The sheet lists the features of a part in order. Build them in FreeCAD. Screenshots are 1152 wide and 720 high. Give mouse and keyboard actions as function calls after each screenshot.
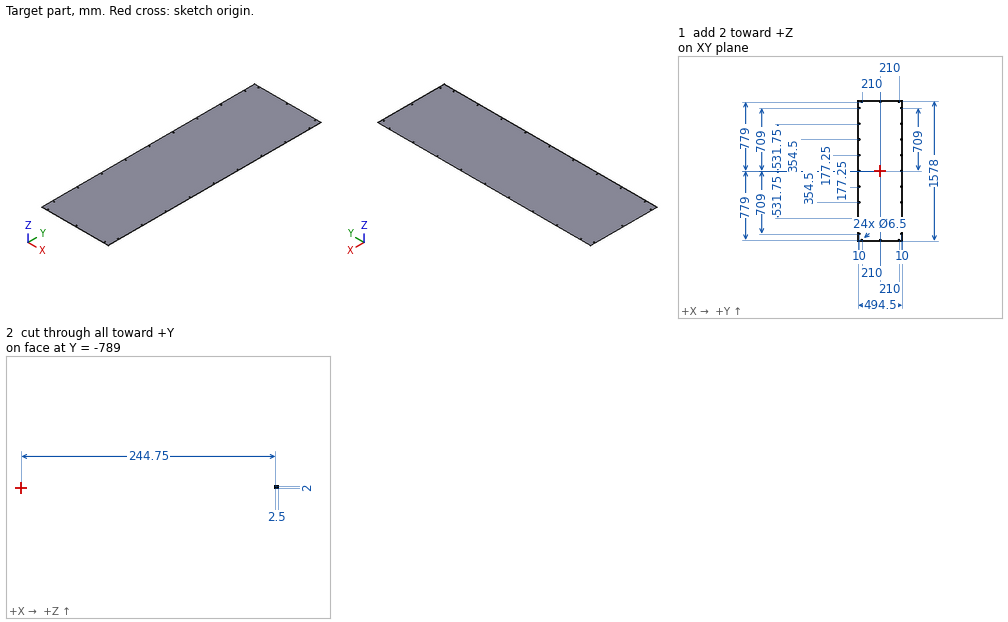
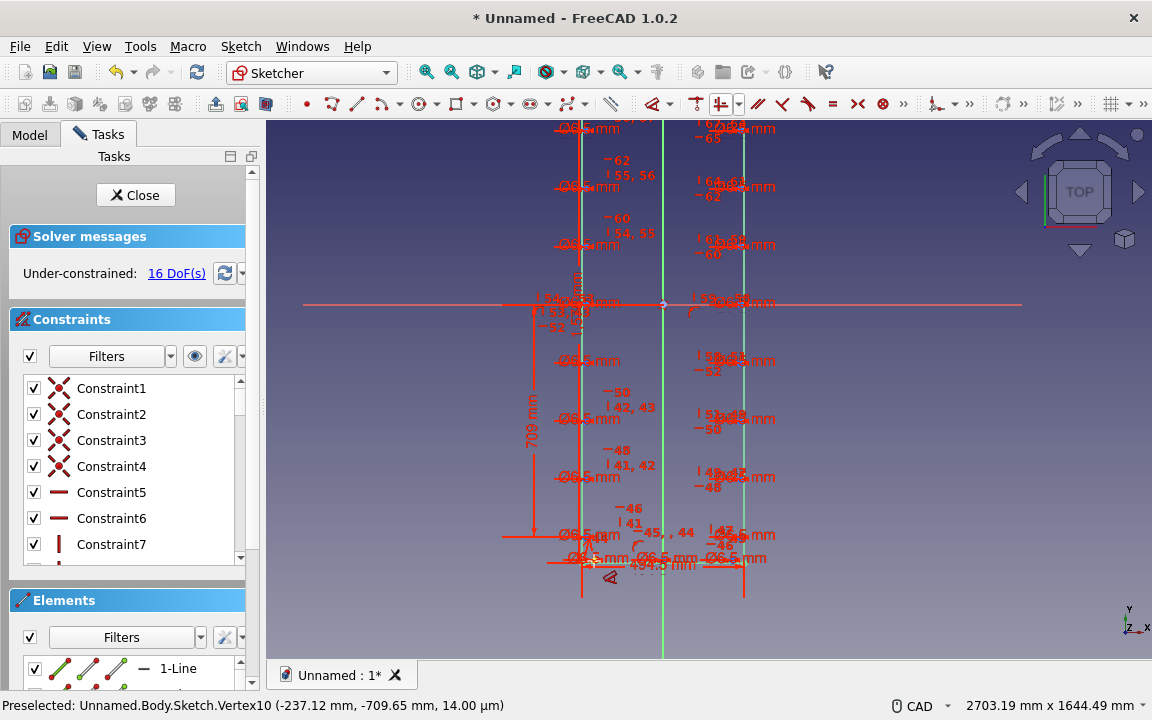
click(594, 560)
click(629, 594)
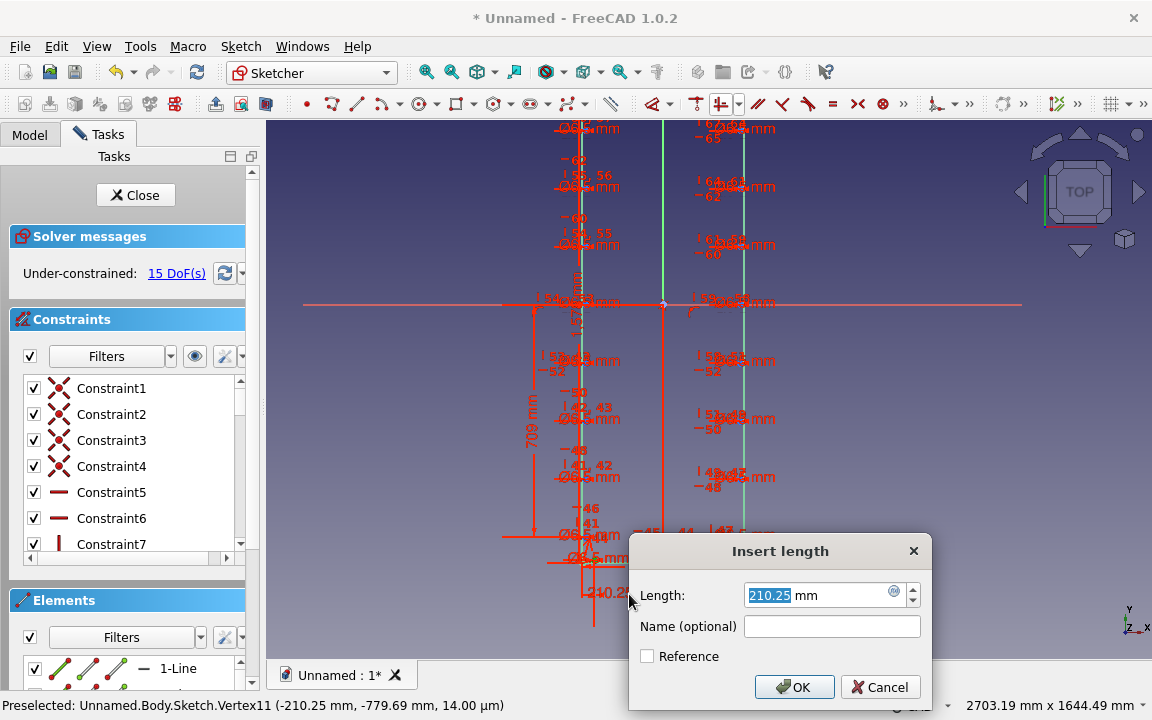
text(210)
key(Return)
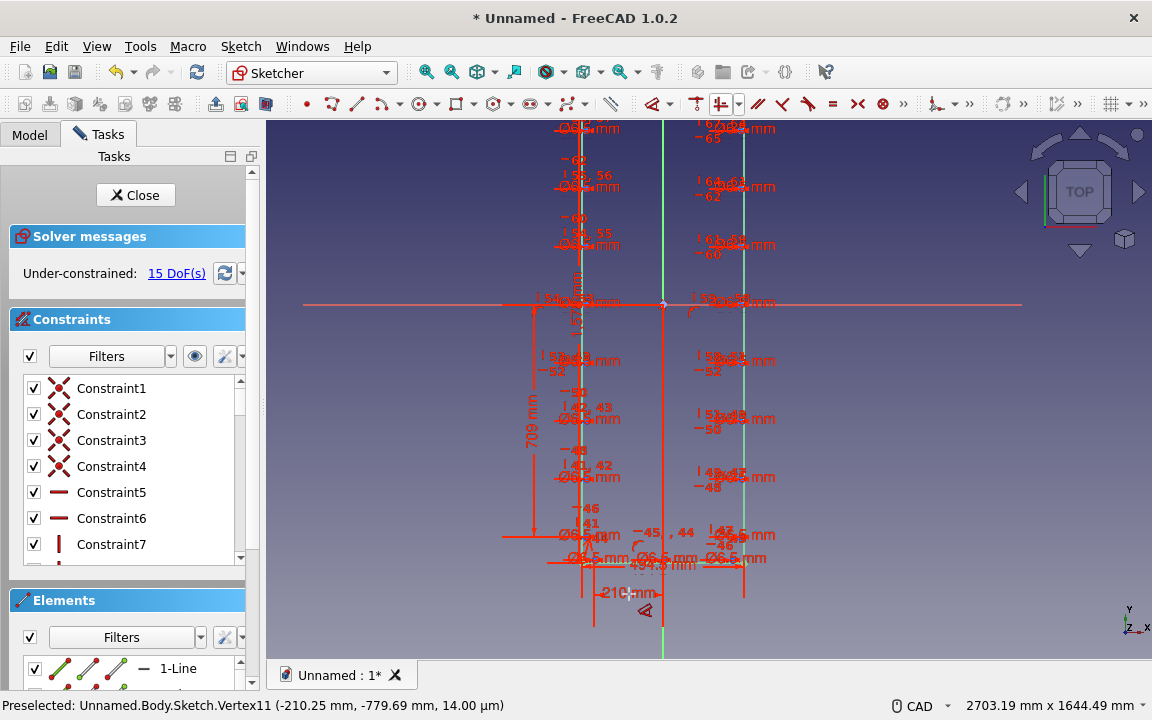
click(594, 560)
click(560, 374)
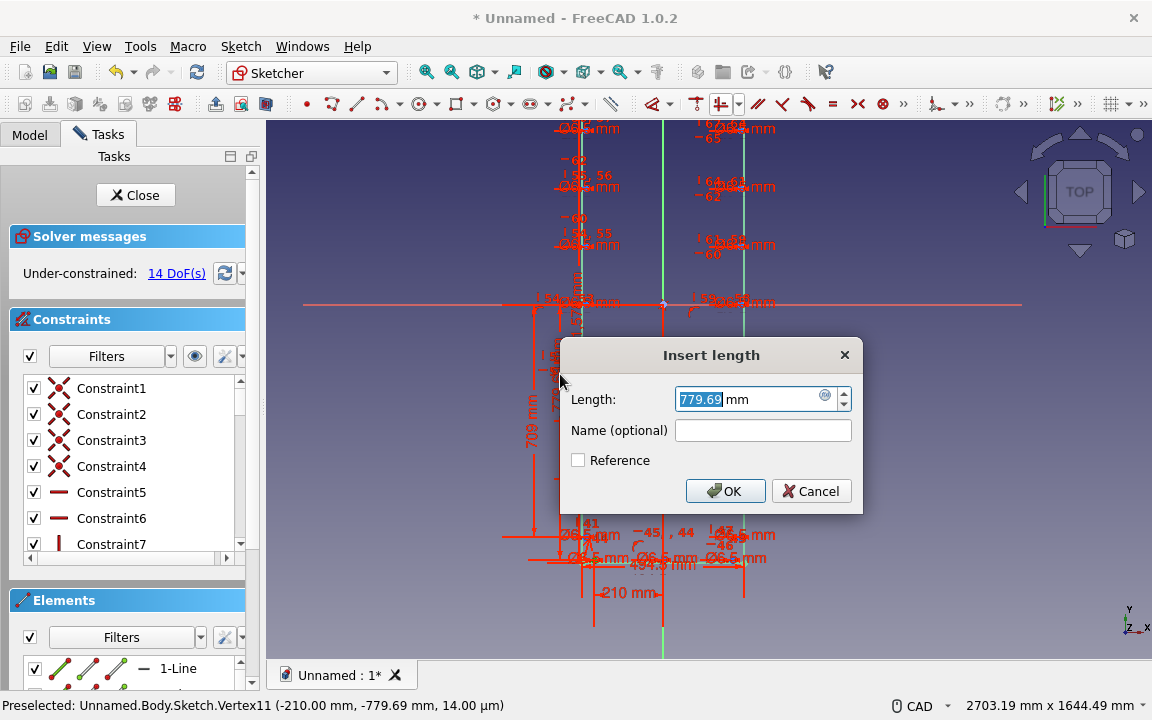
text(779)
key(Return)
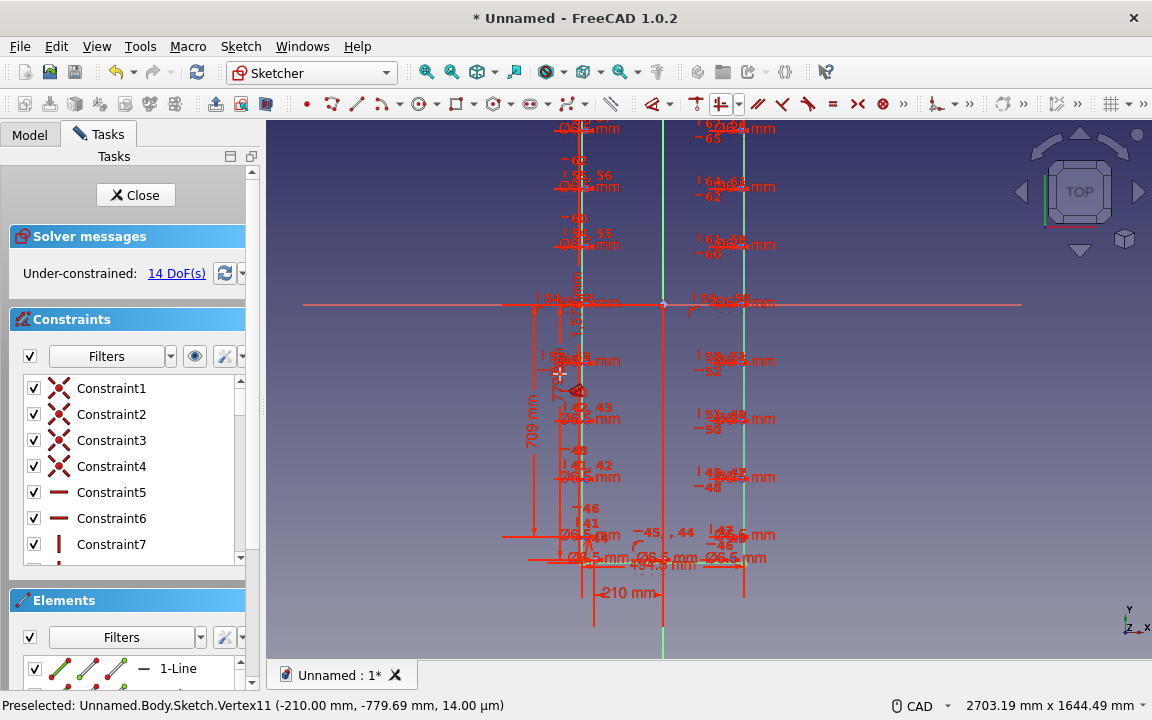
click(732, 560)
click(714, 594)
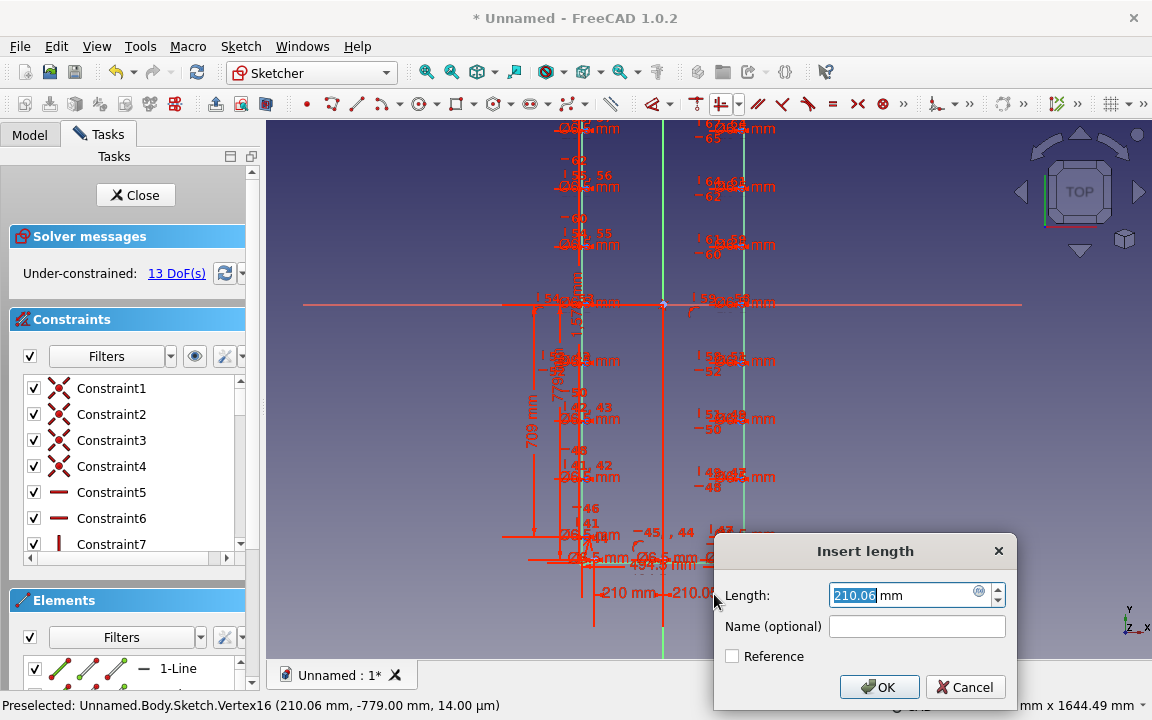
text(210)
key(Return)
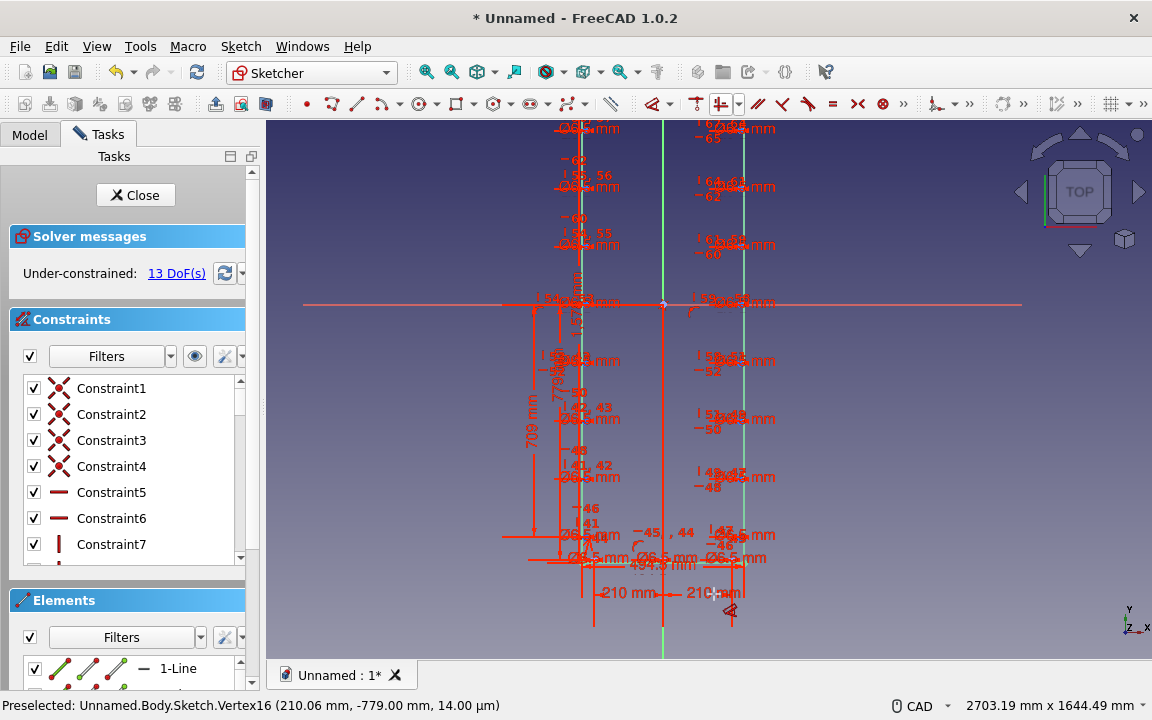
scroll(594, 562, down, 2)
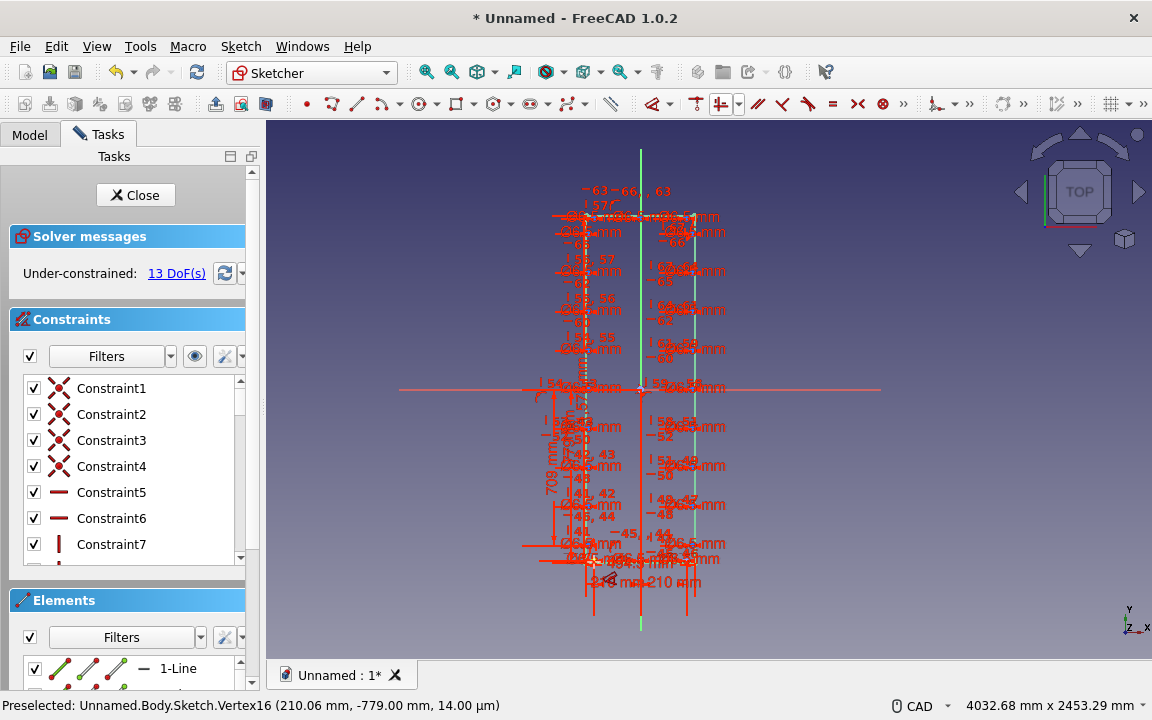
click(588, 234)
click(554, 312)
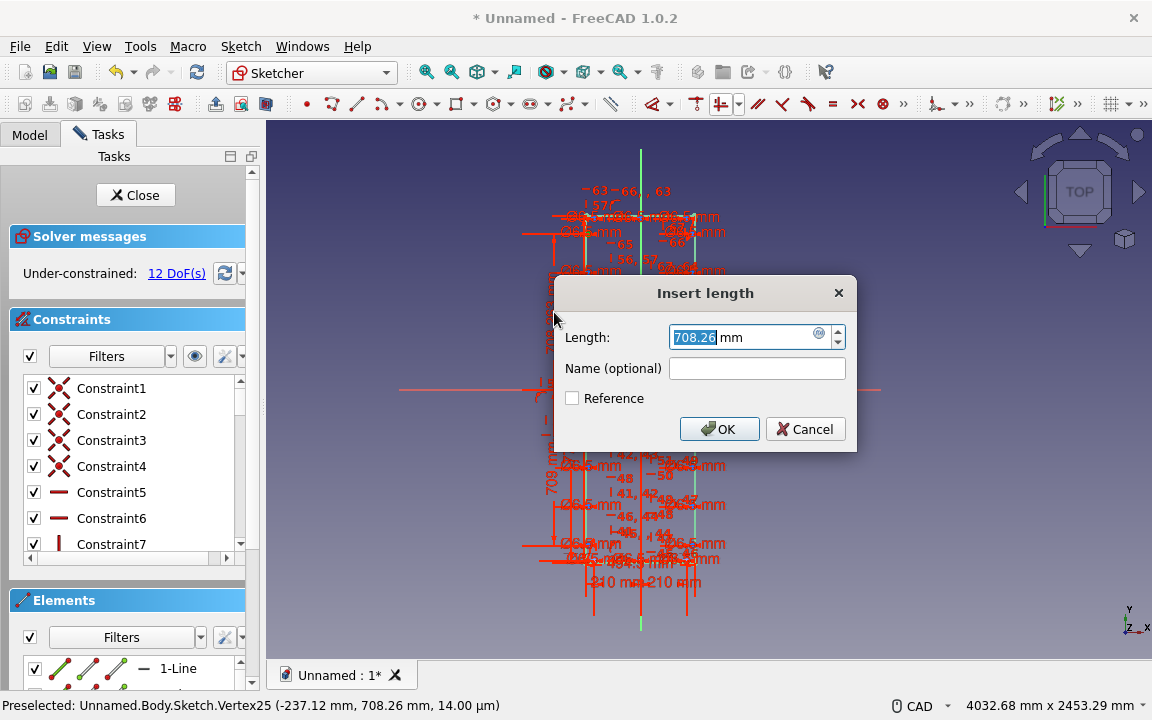
text(709)
key(Return)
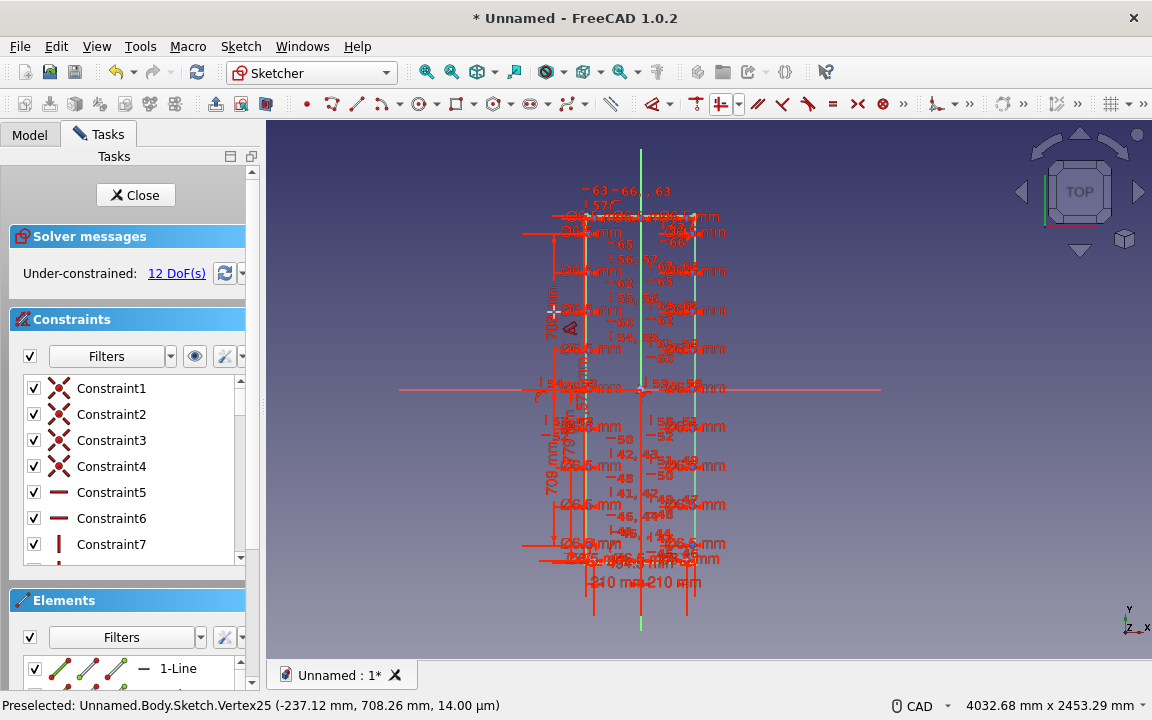
scroll(594, 219, up, 2)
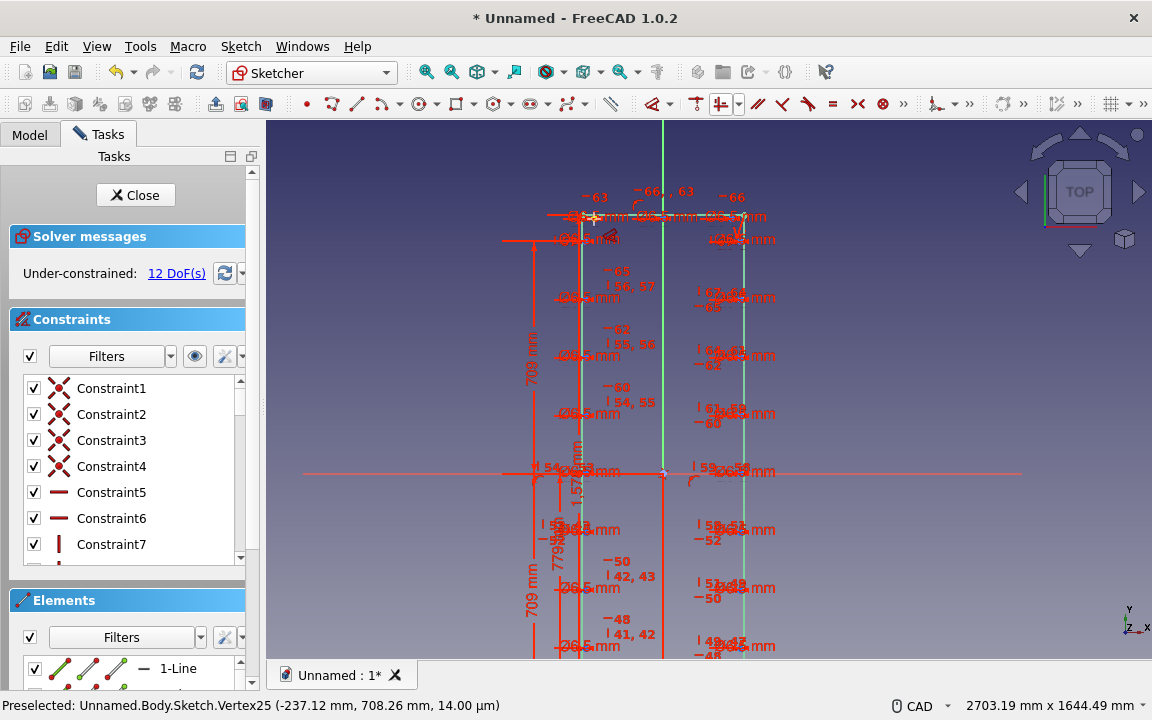
click(594, 219)
click(629, 185)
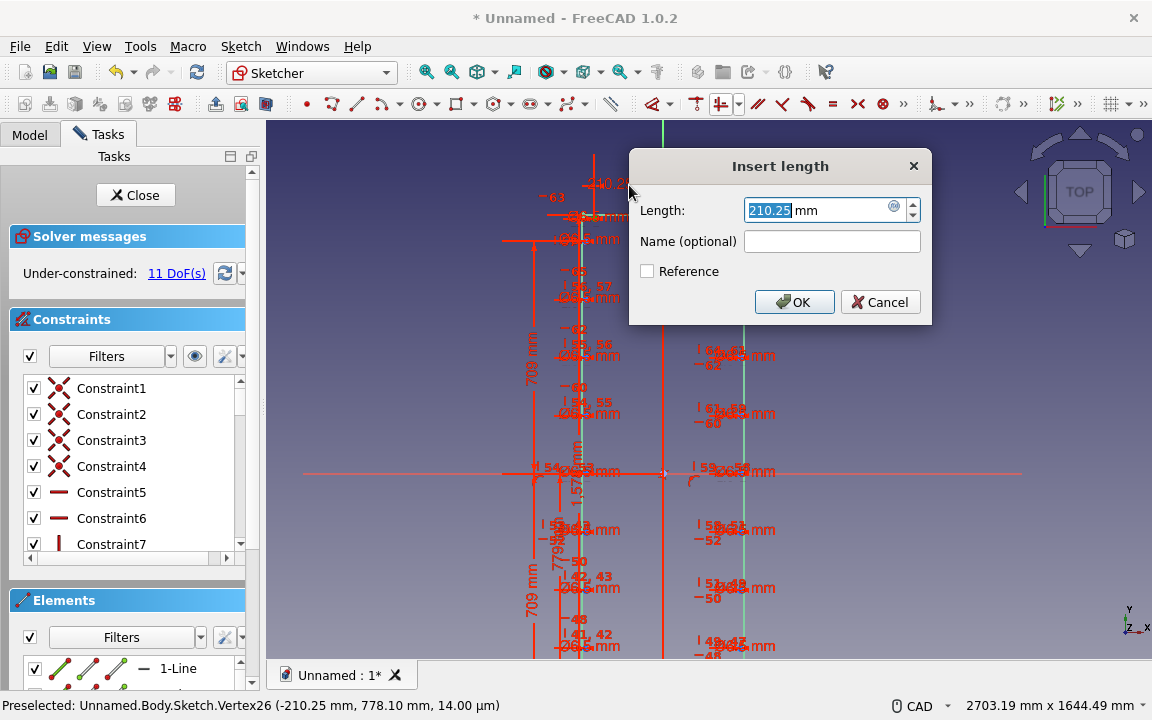
text(210)
key(Return)